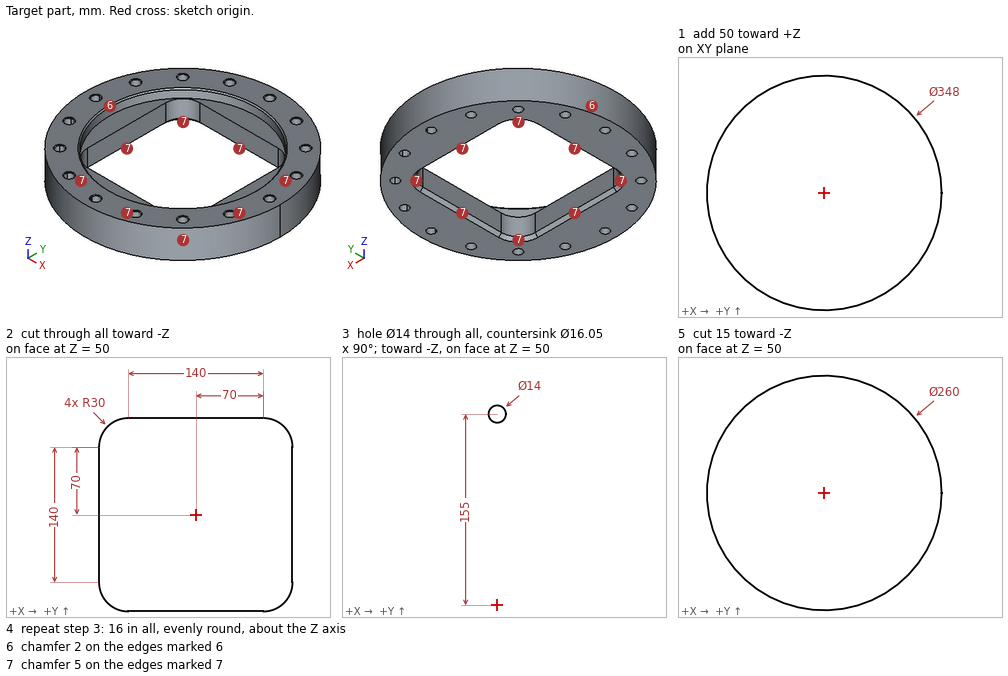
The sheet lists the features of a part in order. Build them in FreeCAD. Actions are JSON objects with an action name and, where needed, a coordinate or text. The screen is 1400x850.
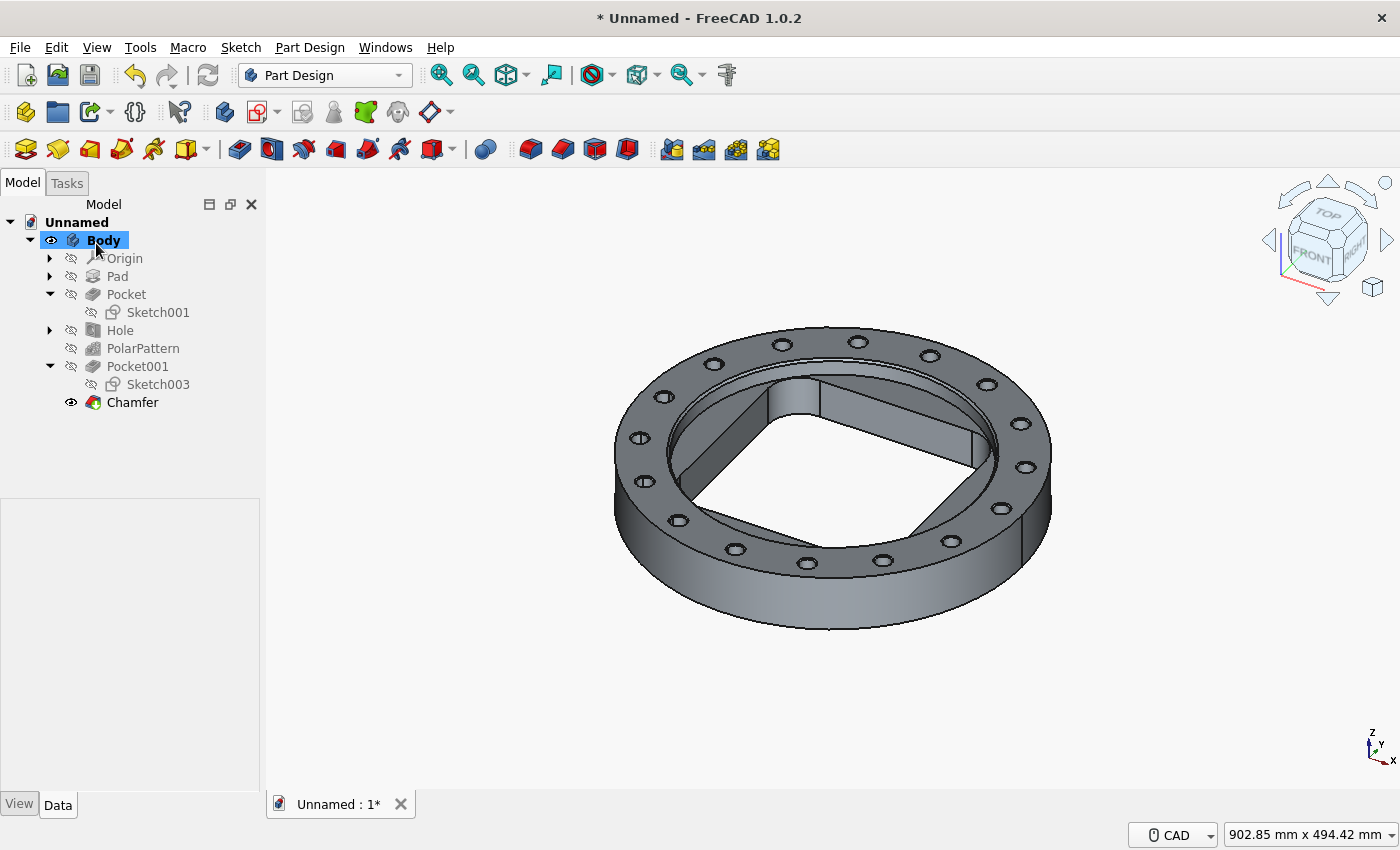
{"action": "key", "text": "0"}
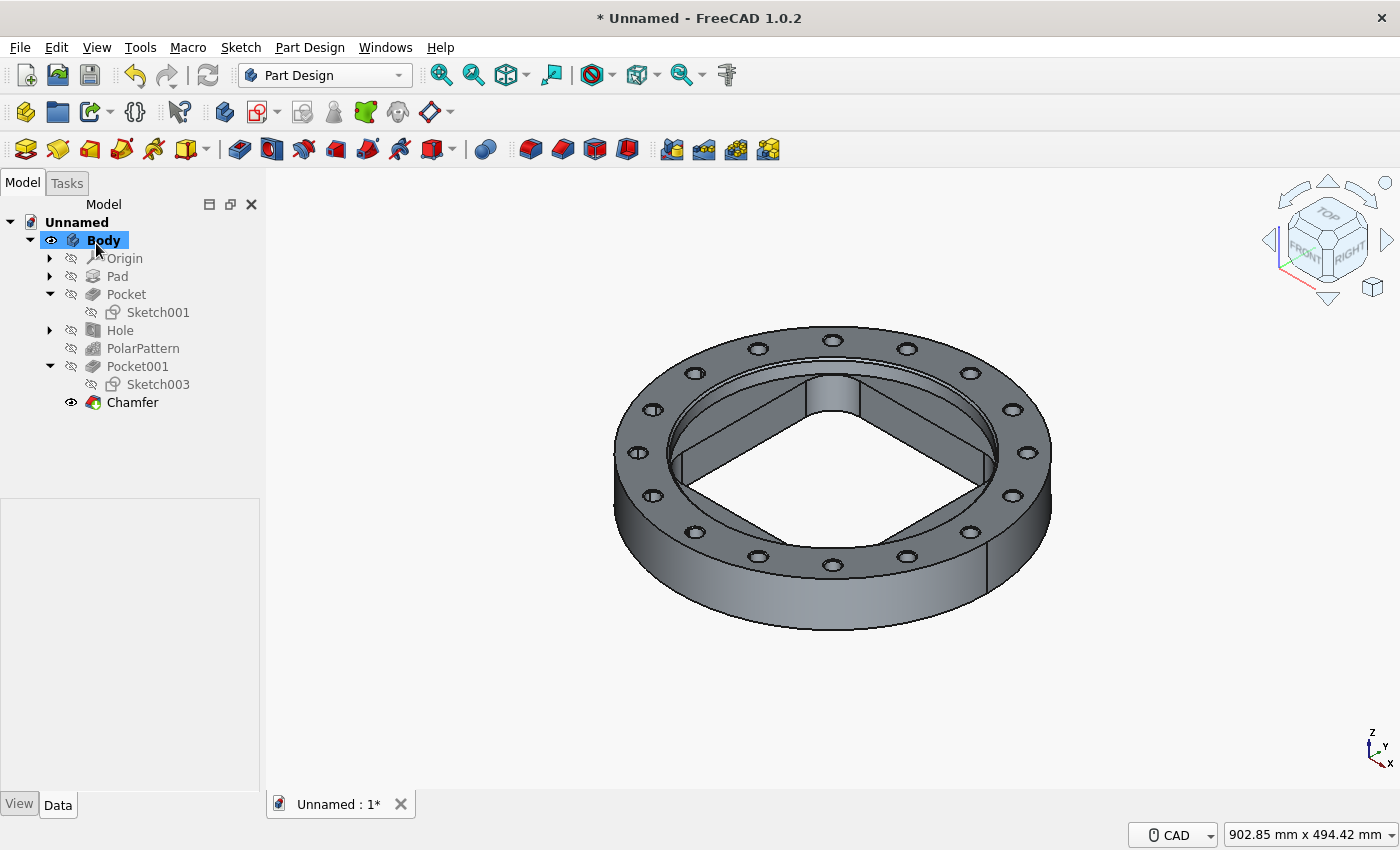
{"action": "key", "text": "2"}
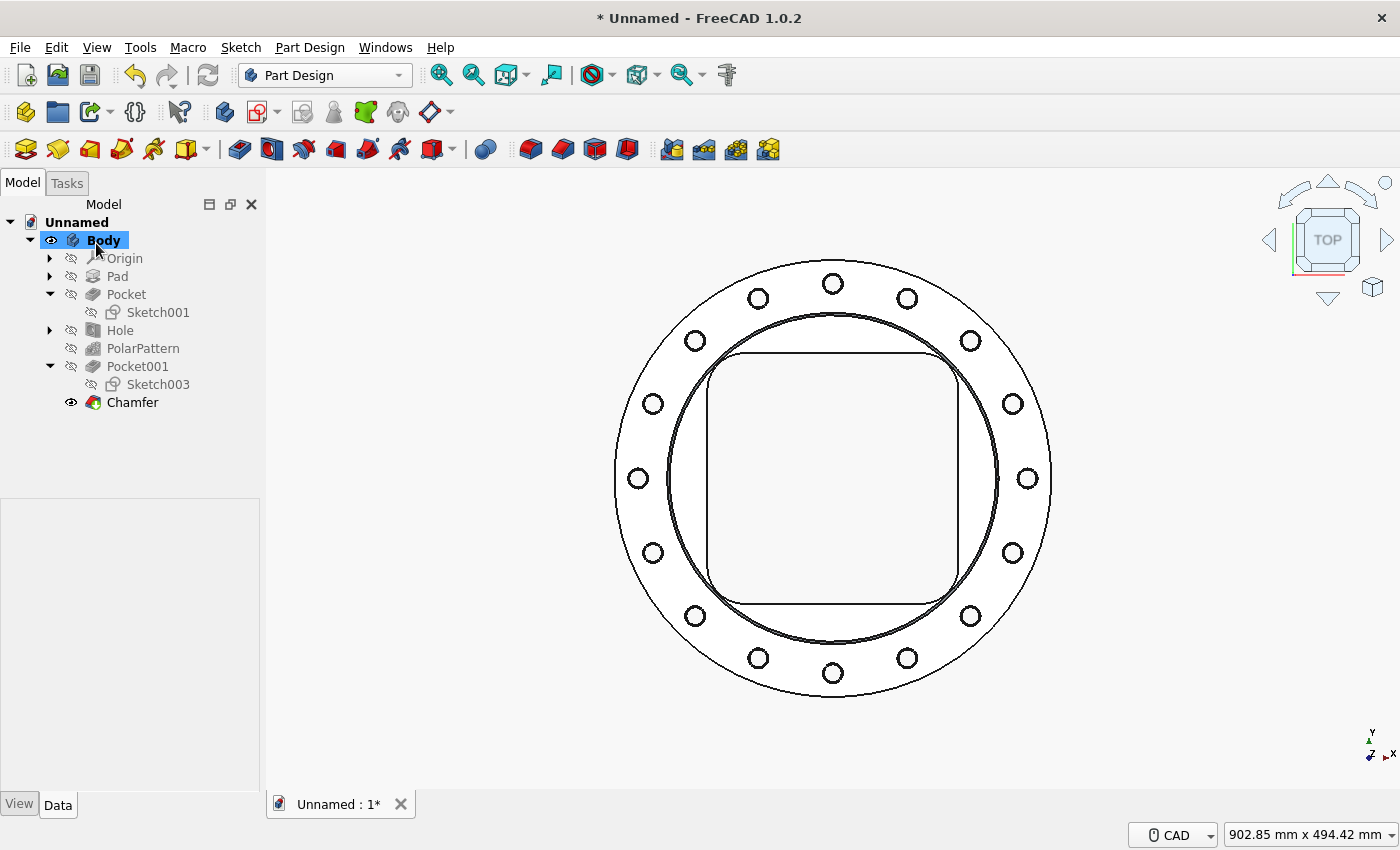
{"action": "key", "text": "1"}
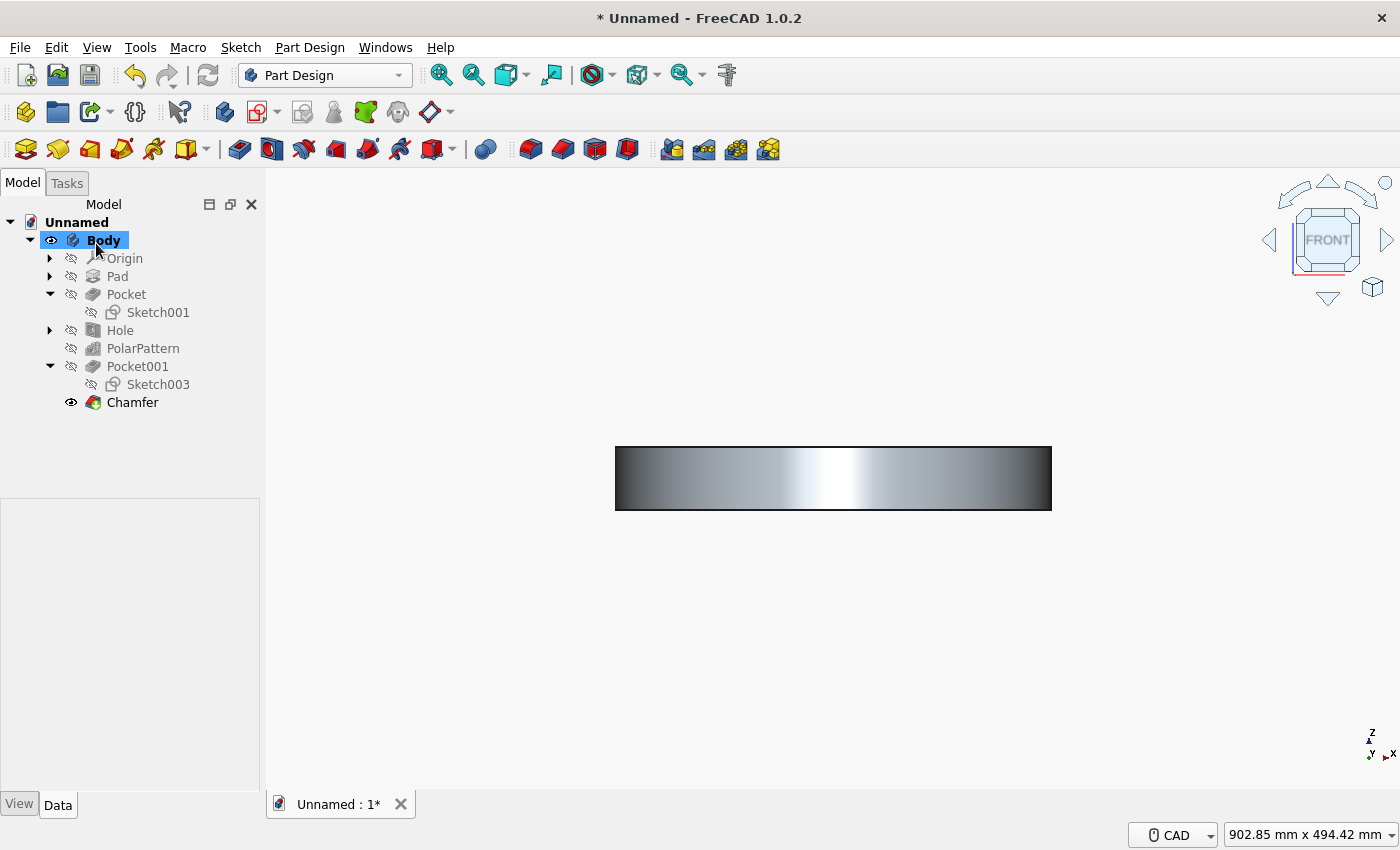
{"action": "left_click", "coordinate": [442, 76]}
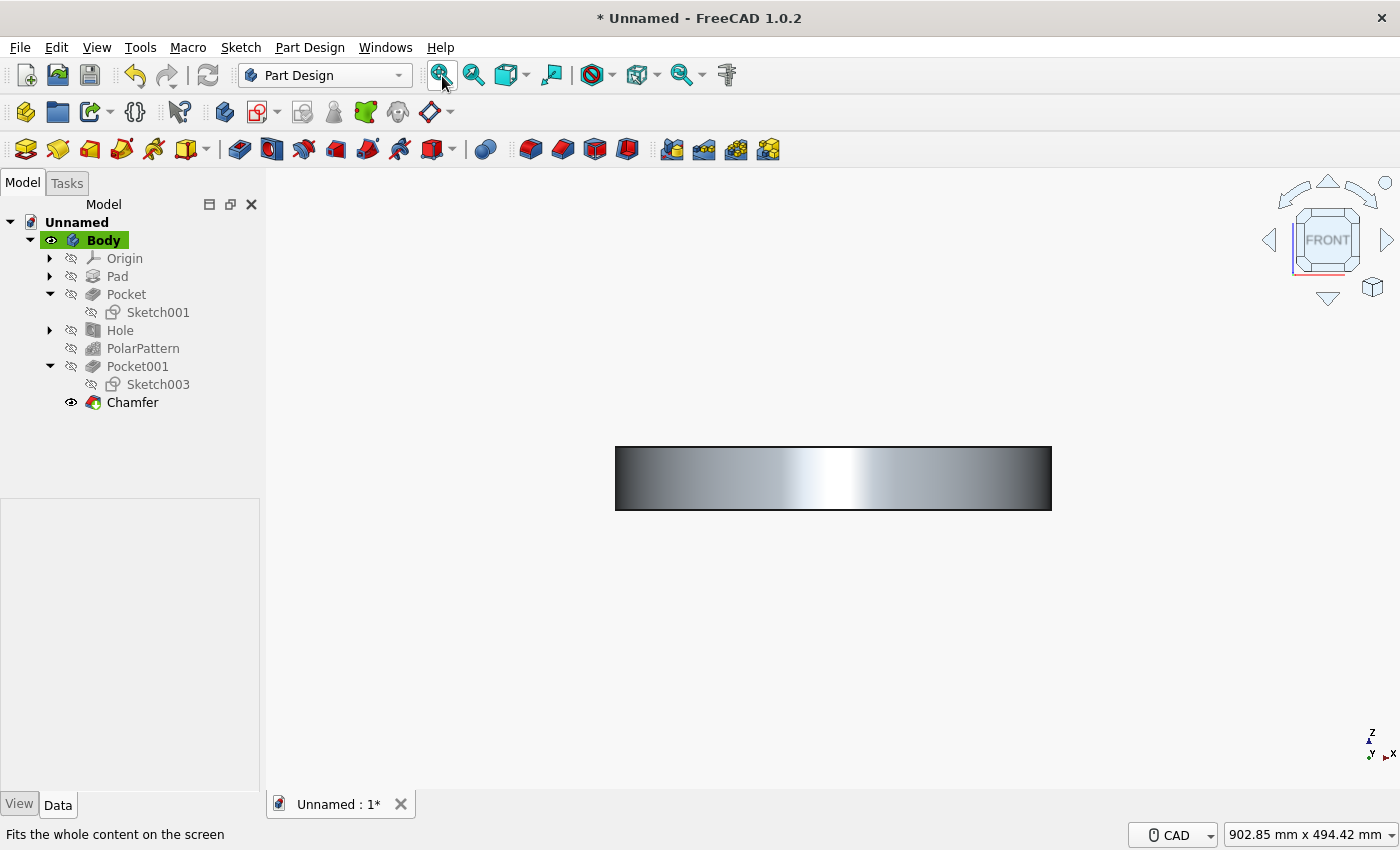
{"action": "key", "text": "3"}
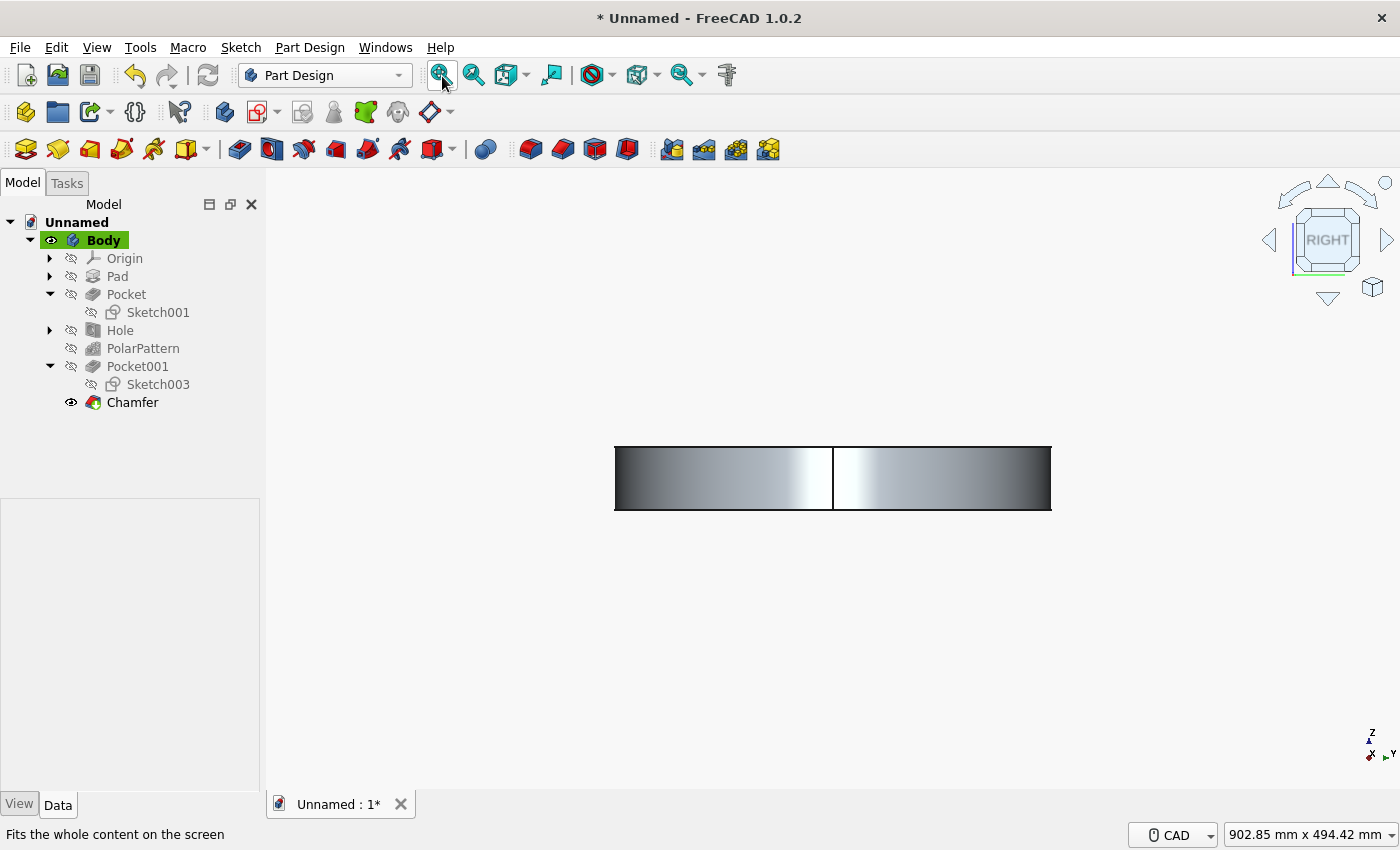
{"action": "left_click", "coordinate": [442, 76]}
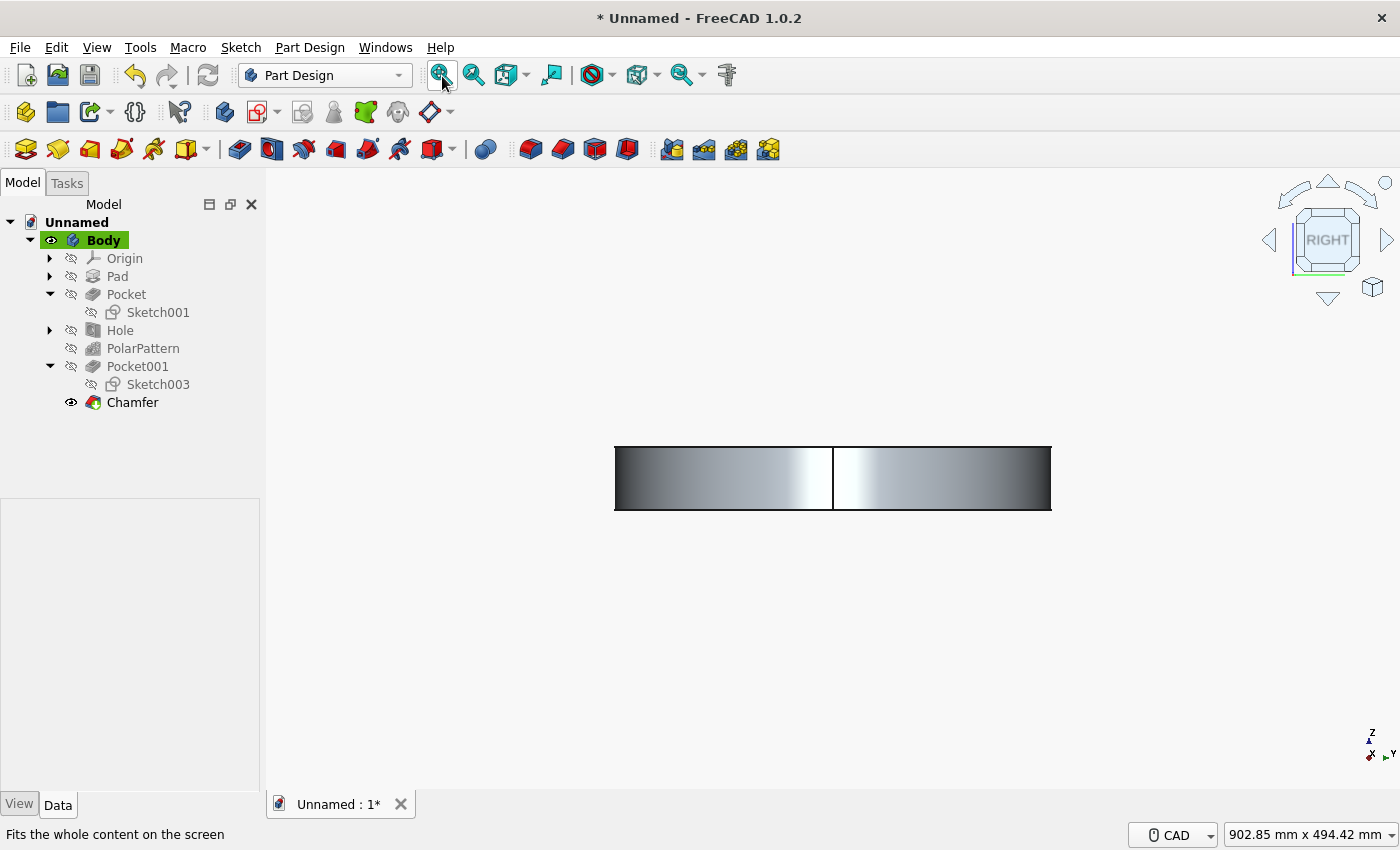
{"action": "key", "text": "5"}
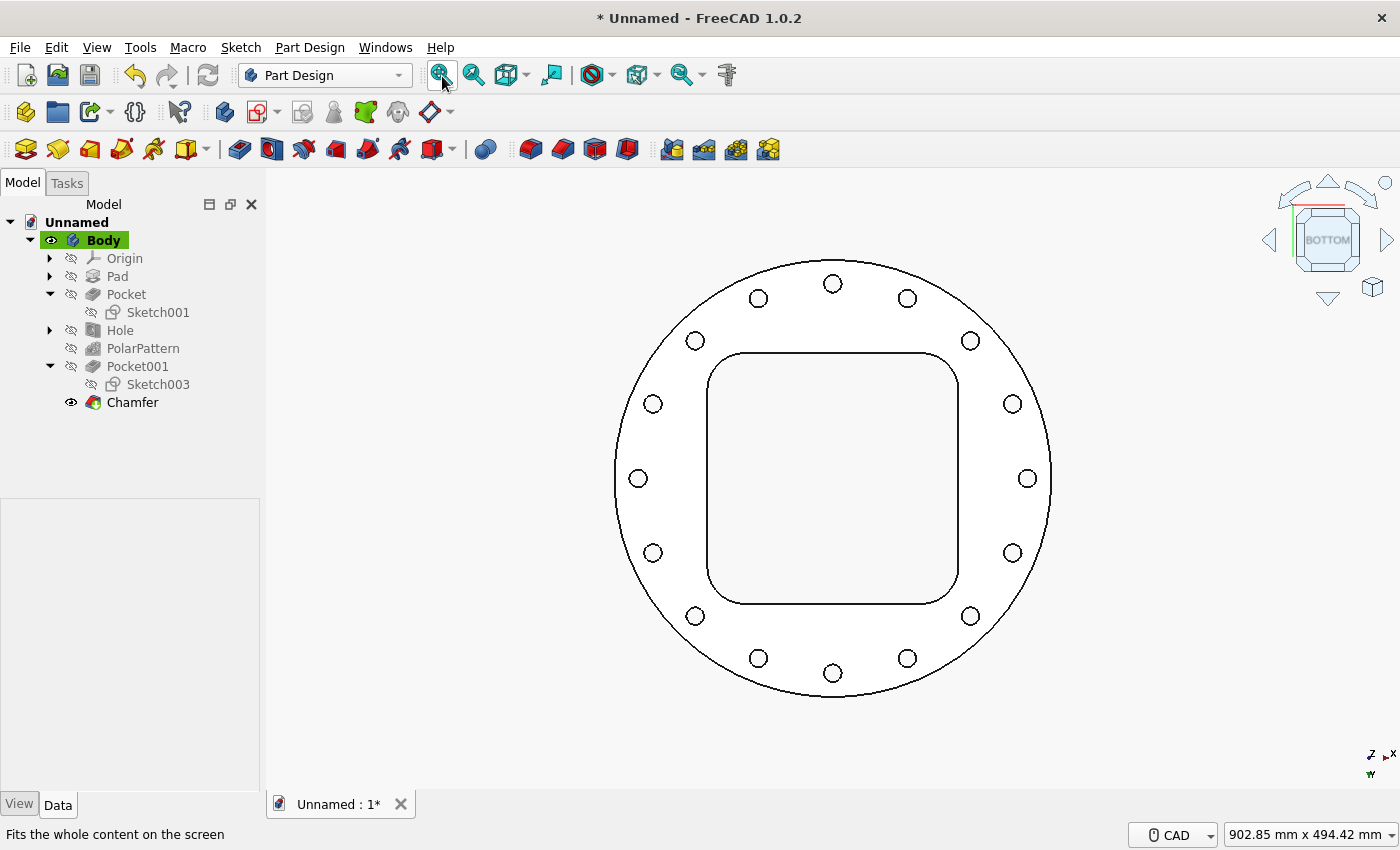
{"action": "left_click", "coordinate": [728, 599]}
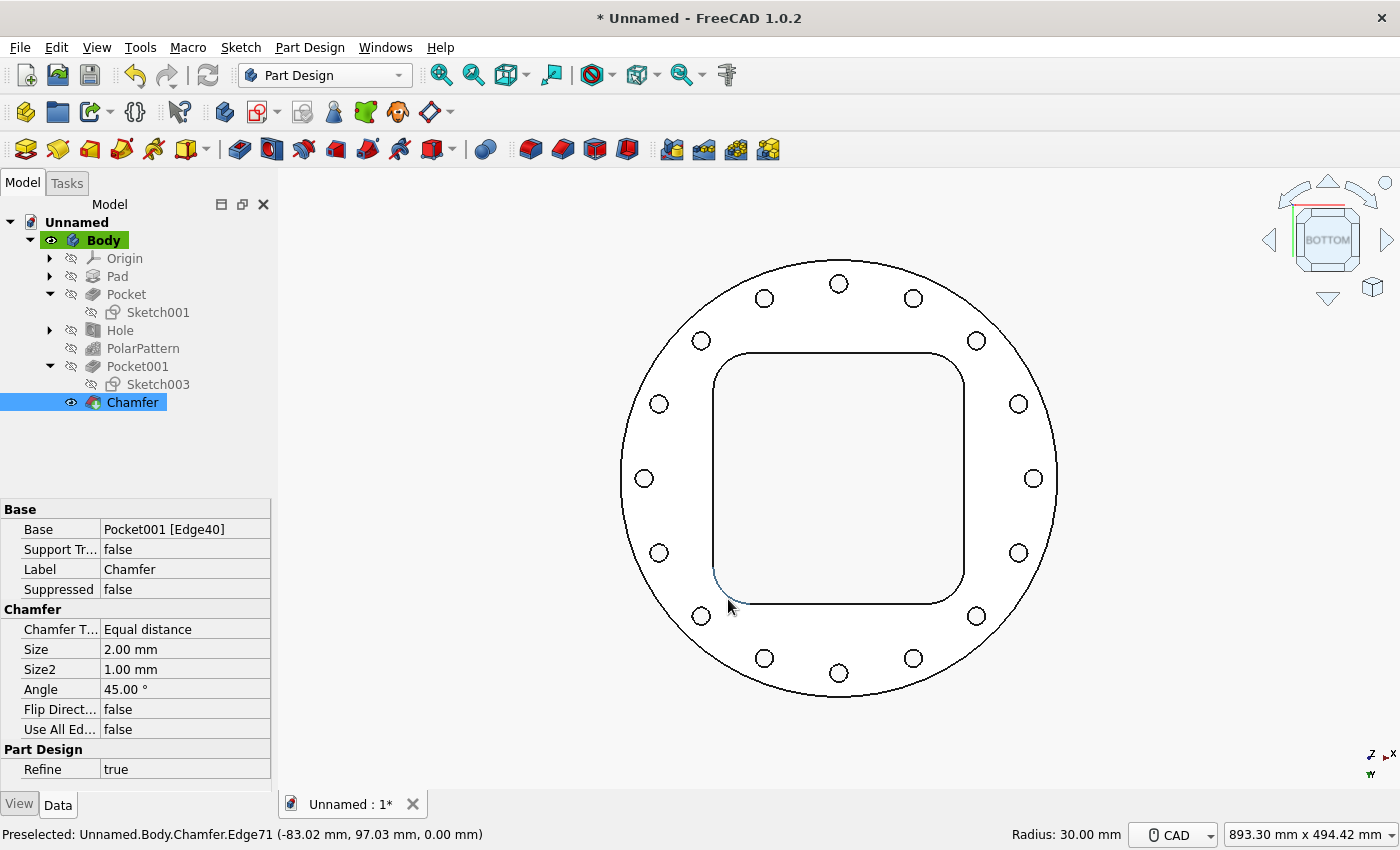
{"action": "left_click", "coordinate": [839, 603], "text": "ctrl"}